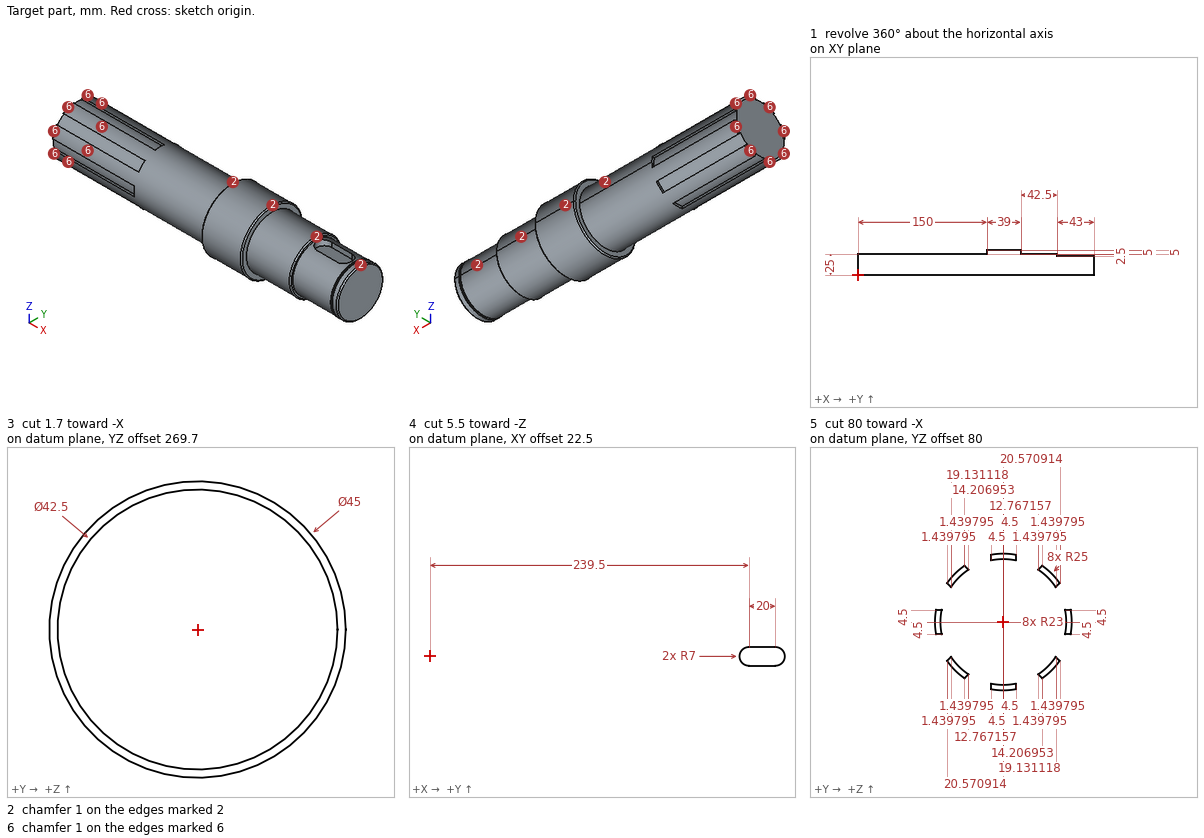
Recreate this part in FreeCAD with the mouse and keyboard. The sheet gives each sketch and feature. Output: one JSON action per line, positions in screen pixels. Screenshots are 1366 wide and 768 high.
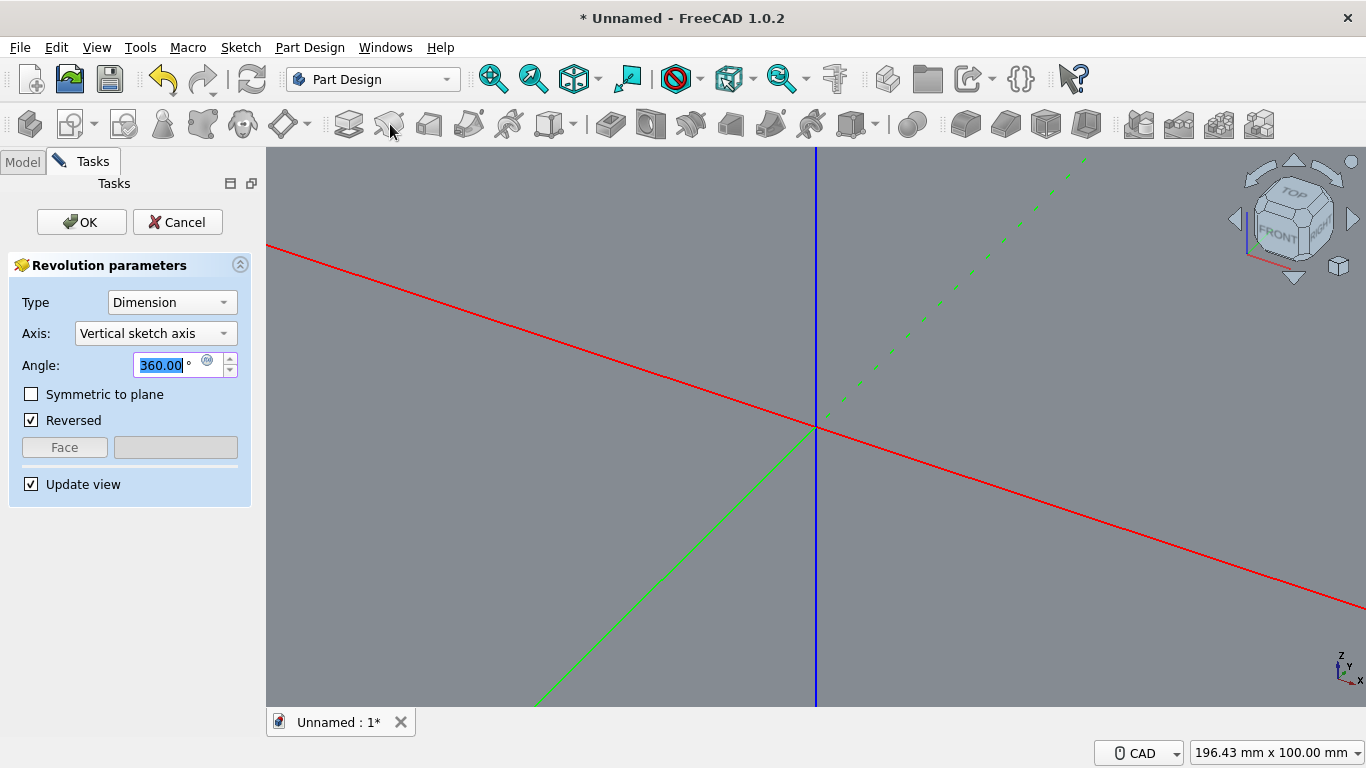
{"action": "left_click", "coordinate": [156, 334]}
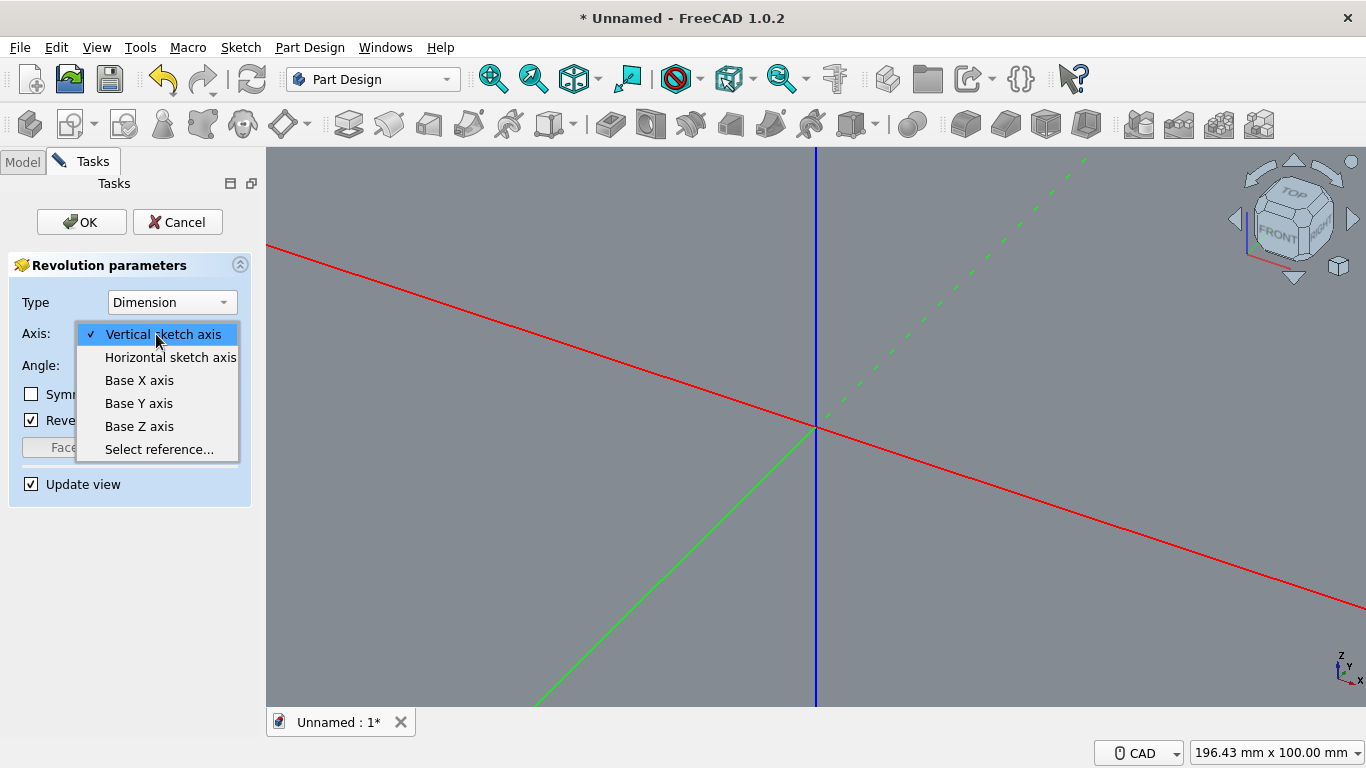
{"action": "left_click", "coordinate": [156, 358]}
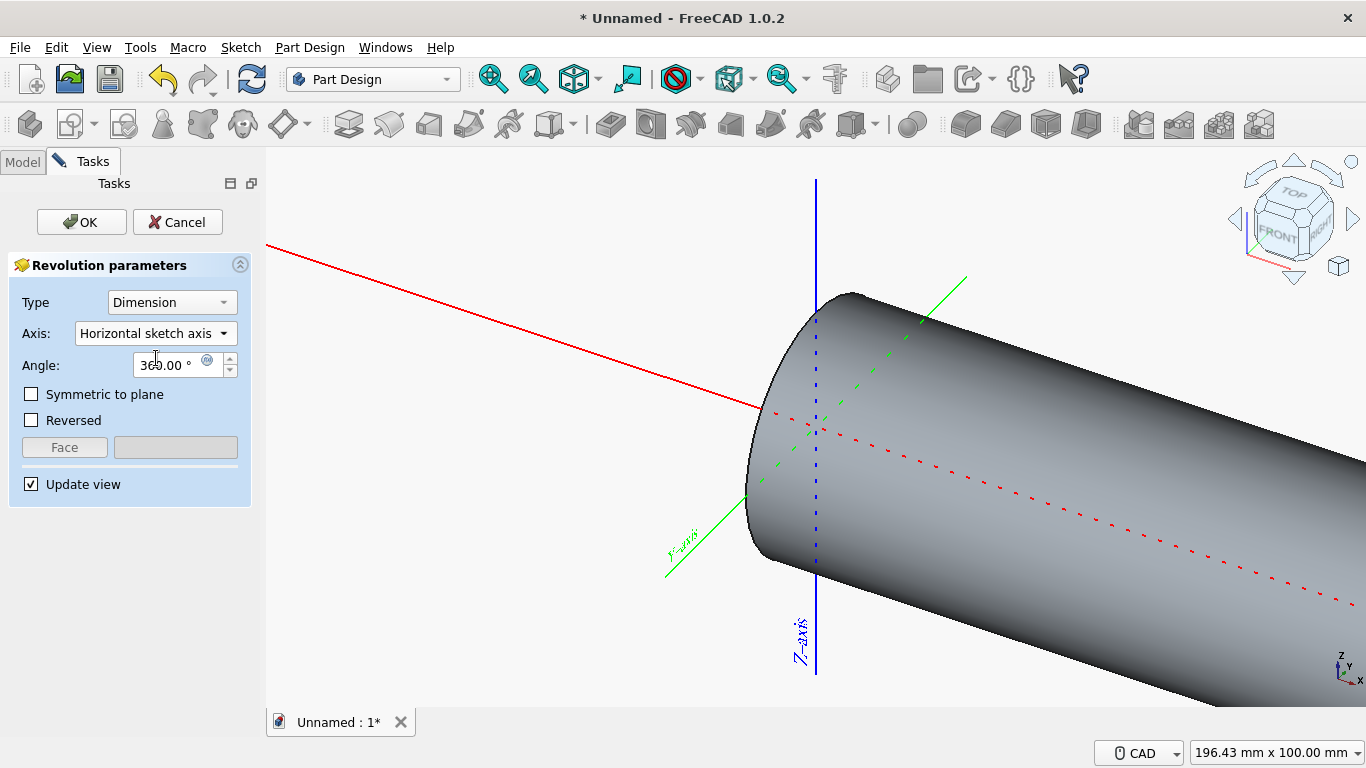
{"action": "left_click", "coordinate": [82, 222]}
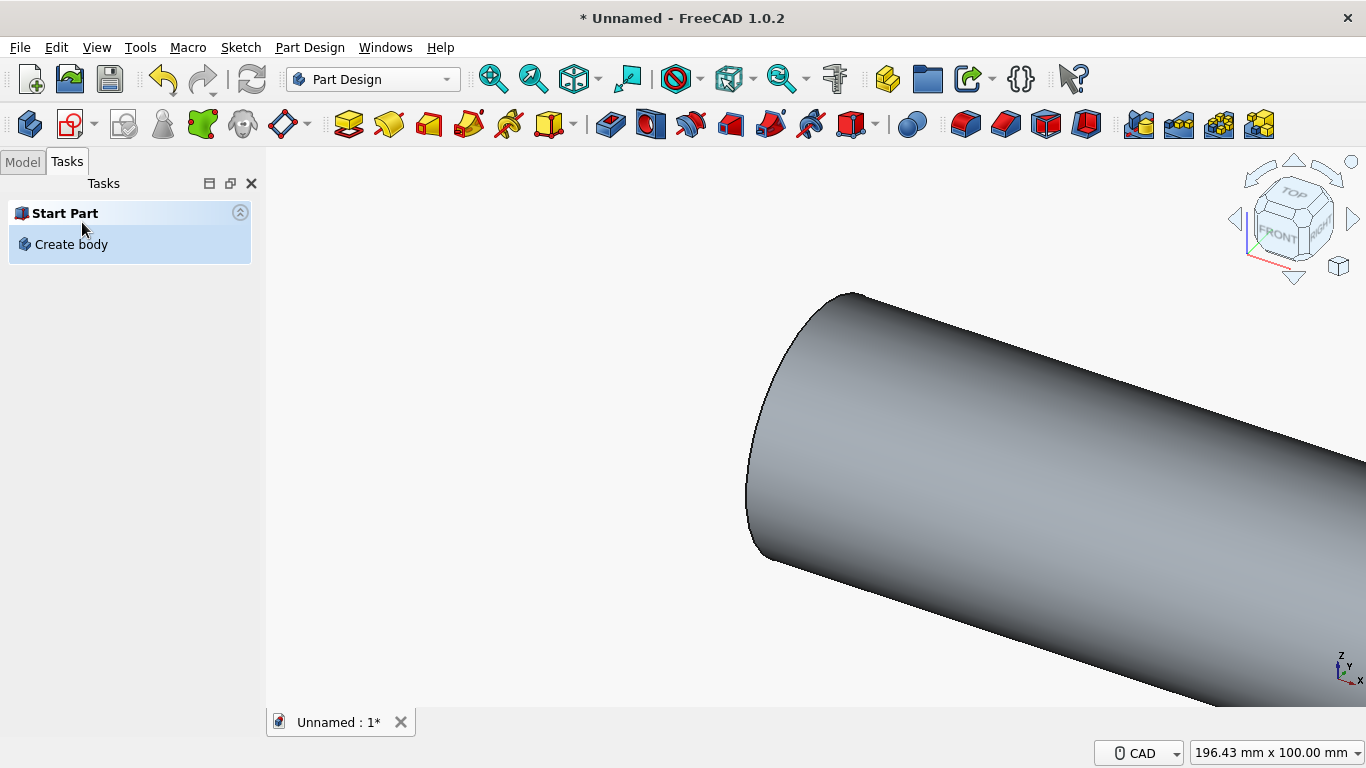
{"action": "left_click", "coordinate": [494, 80]}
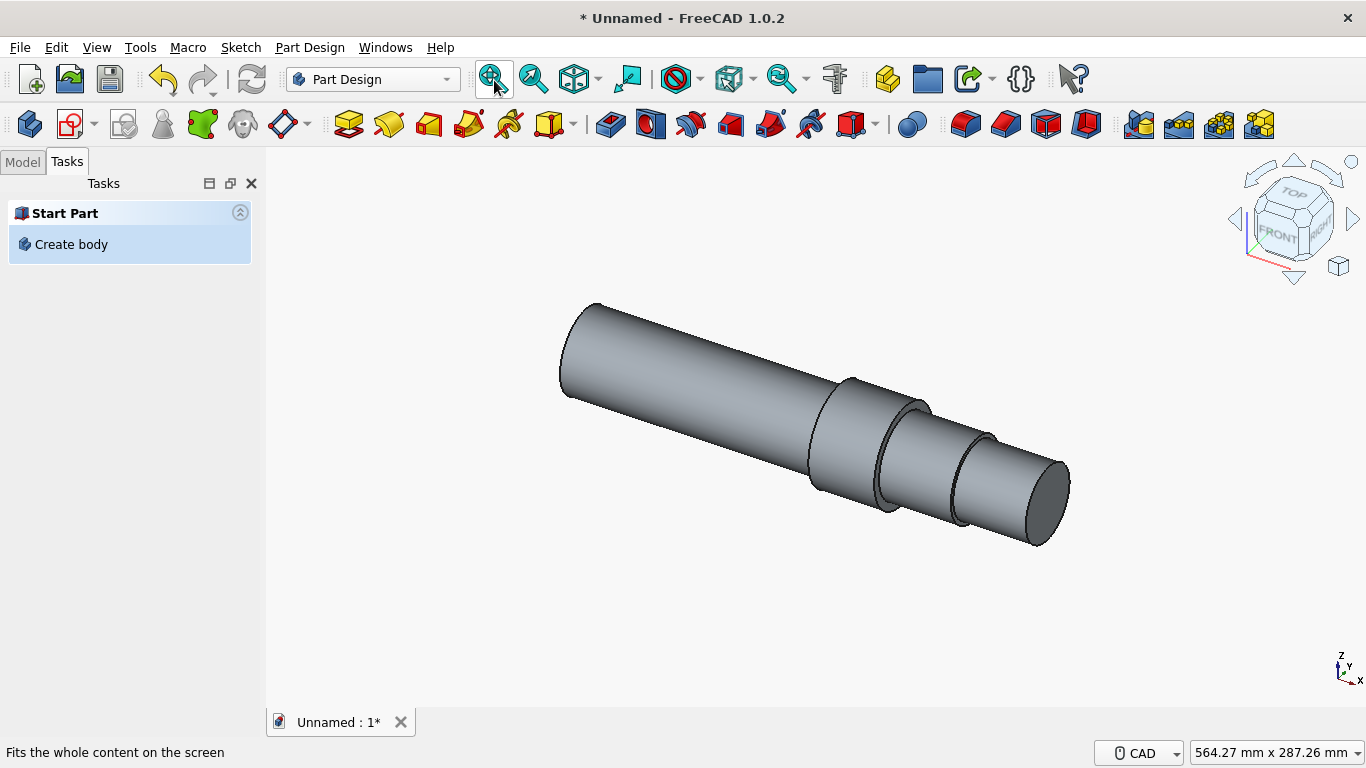
{"action": "left_click", "coordinate": [1026, 525]}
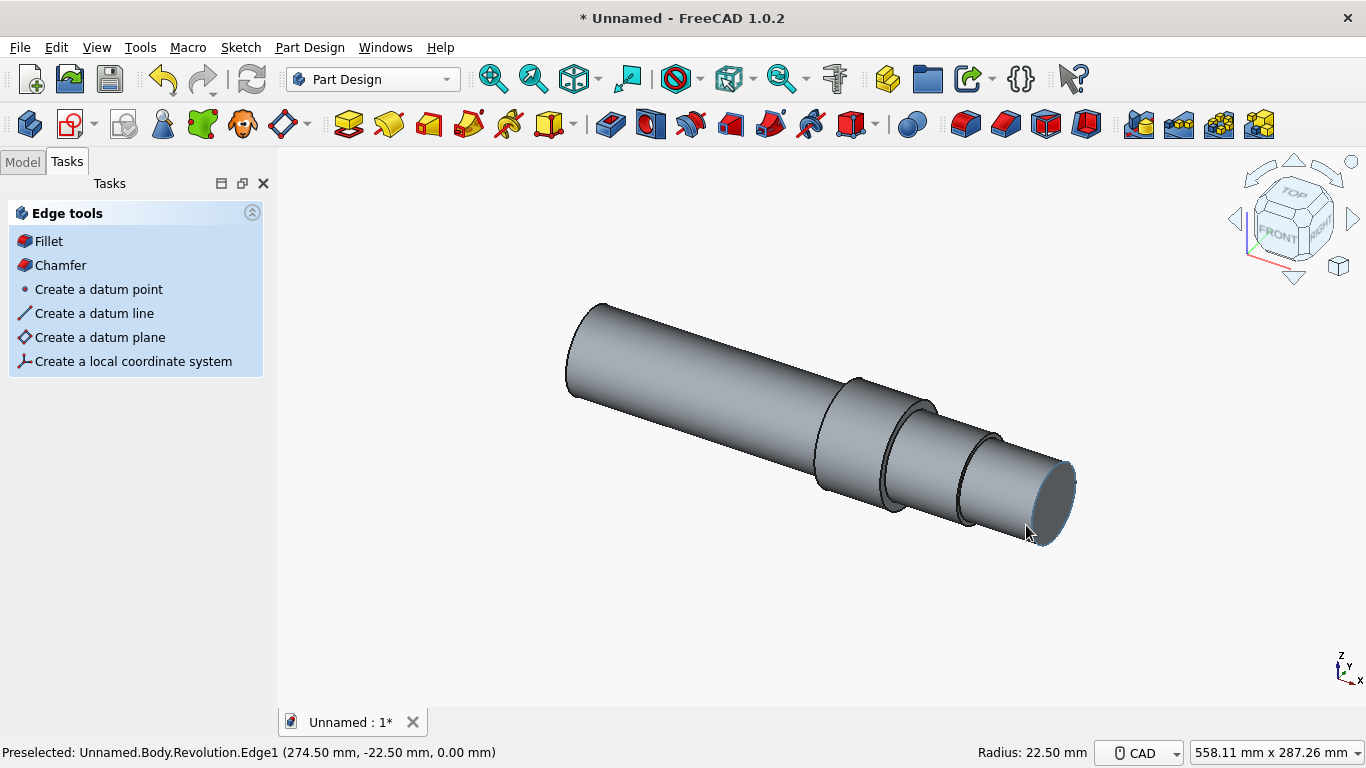
{"action": "left_click", "coordinate": [957, 503], "text": "ctrl"}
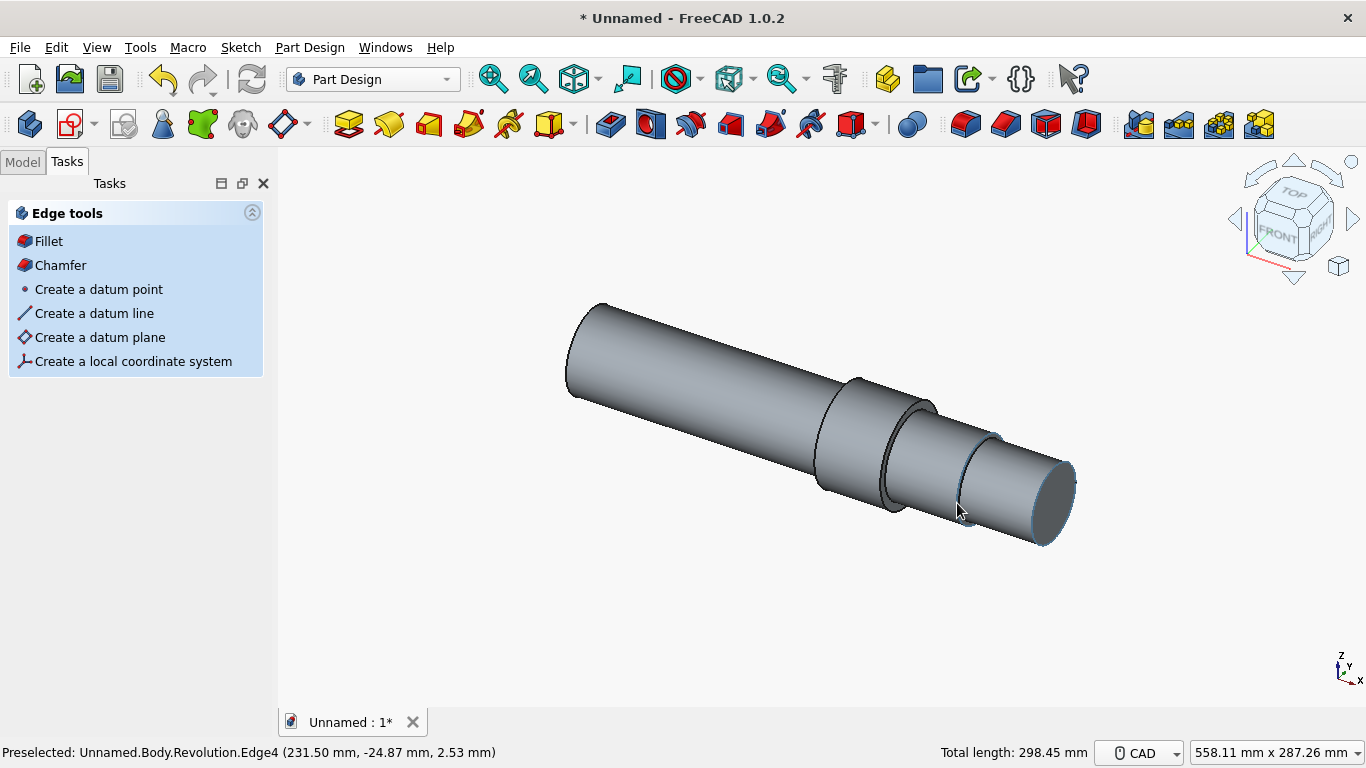
{"action": "left_click", "coordinate": [880, 484], "text": "ctrl"}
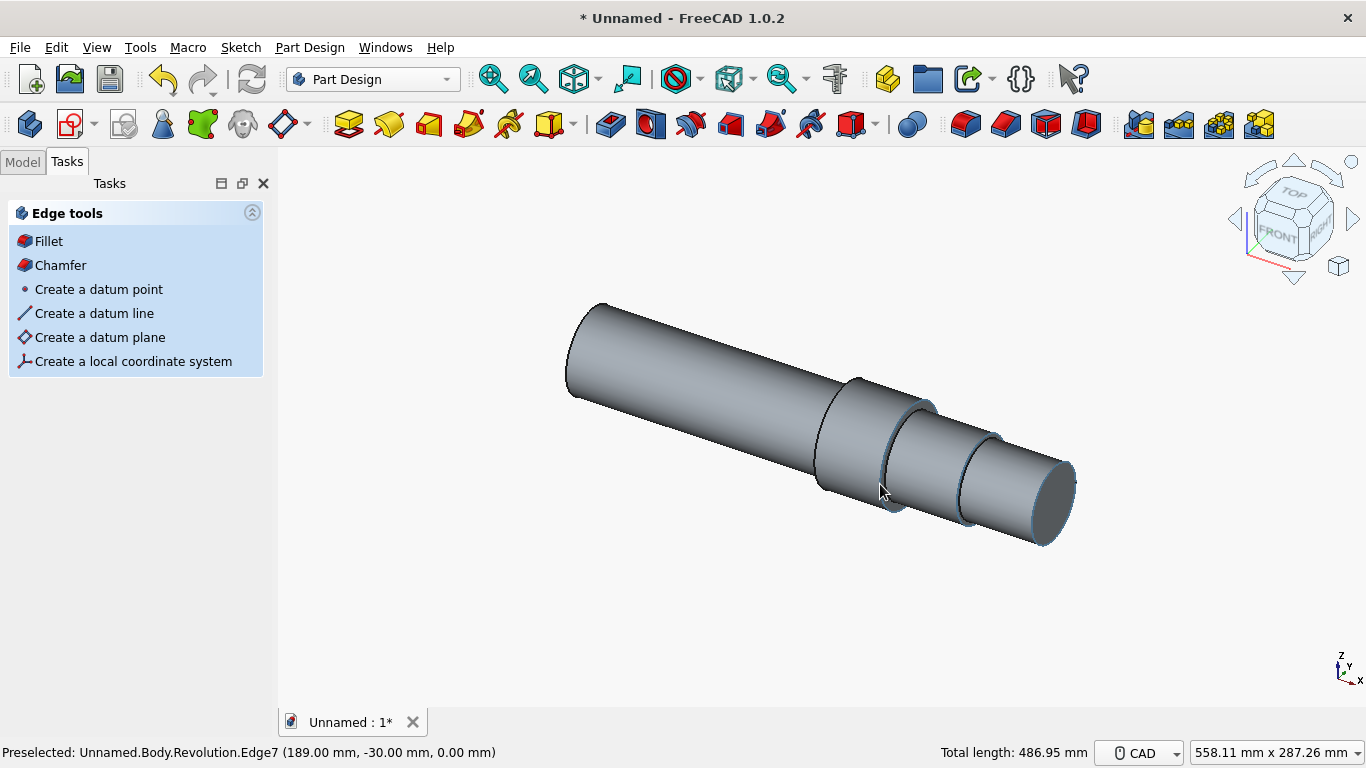
{"action": "key", "text": "0"}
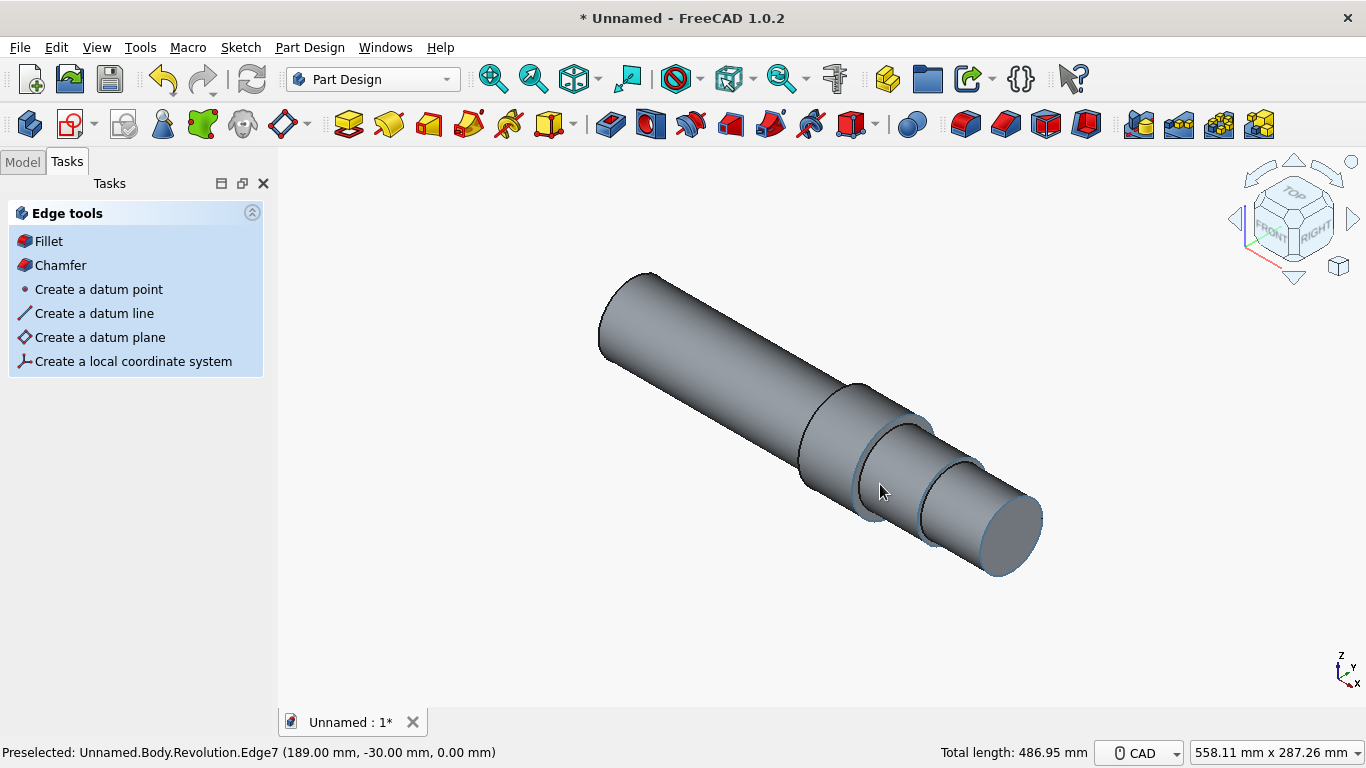
{"action": "key", "text": "2"}